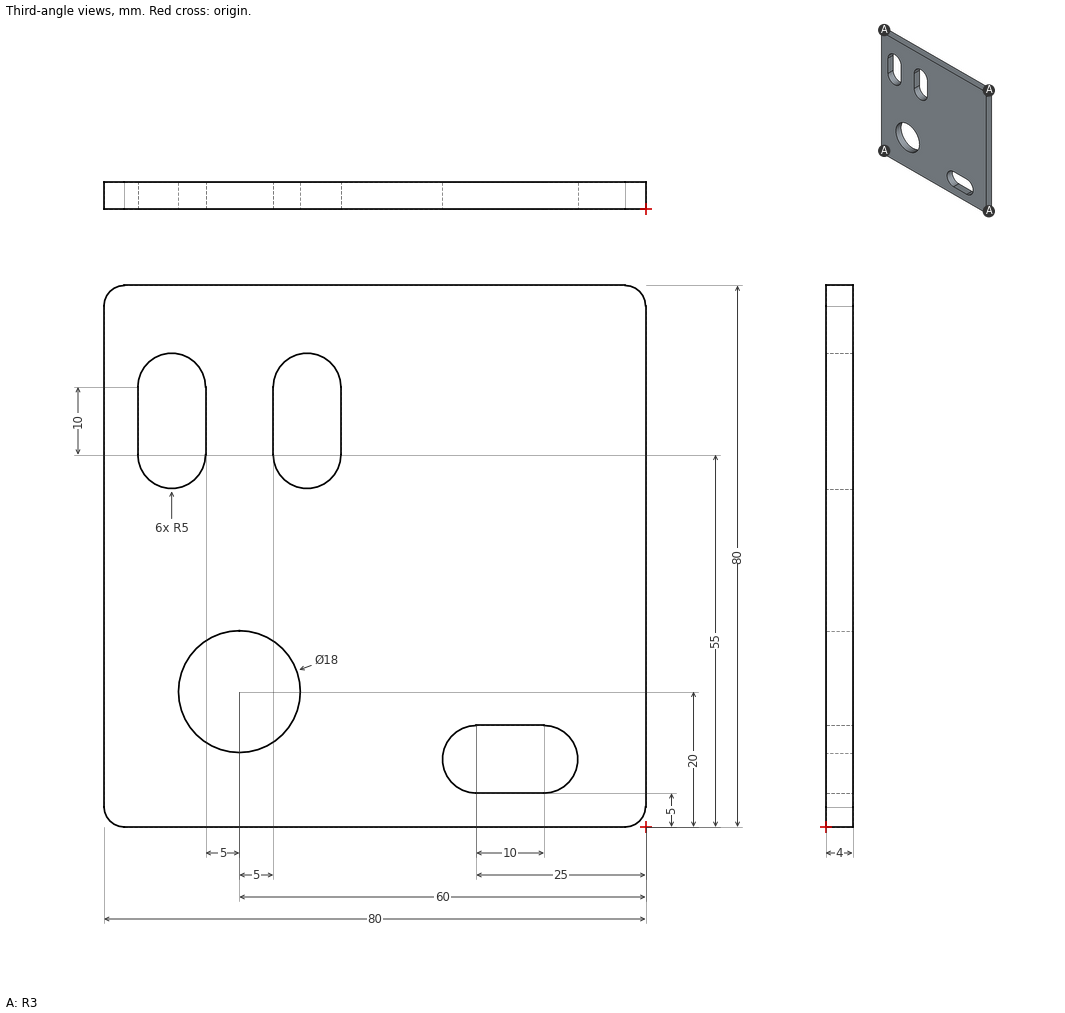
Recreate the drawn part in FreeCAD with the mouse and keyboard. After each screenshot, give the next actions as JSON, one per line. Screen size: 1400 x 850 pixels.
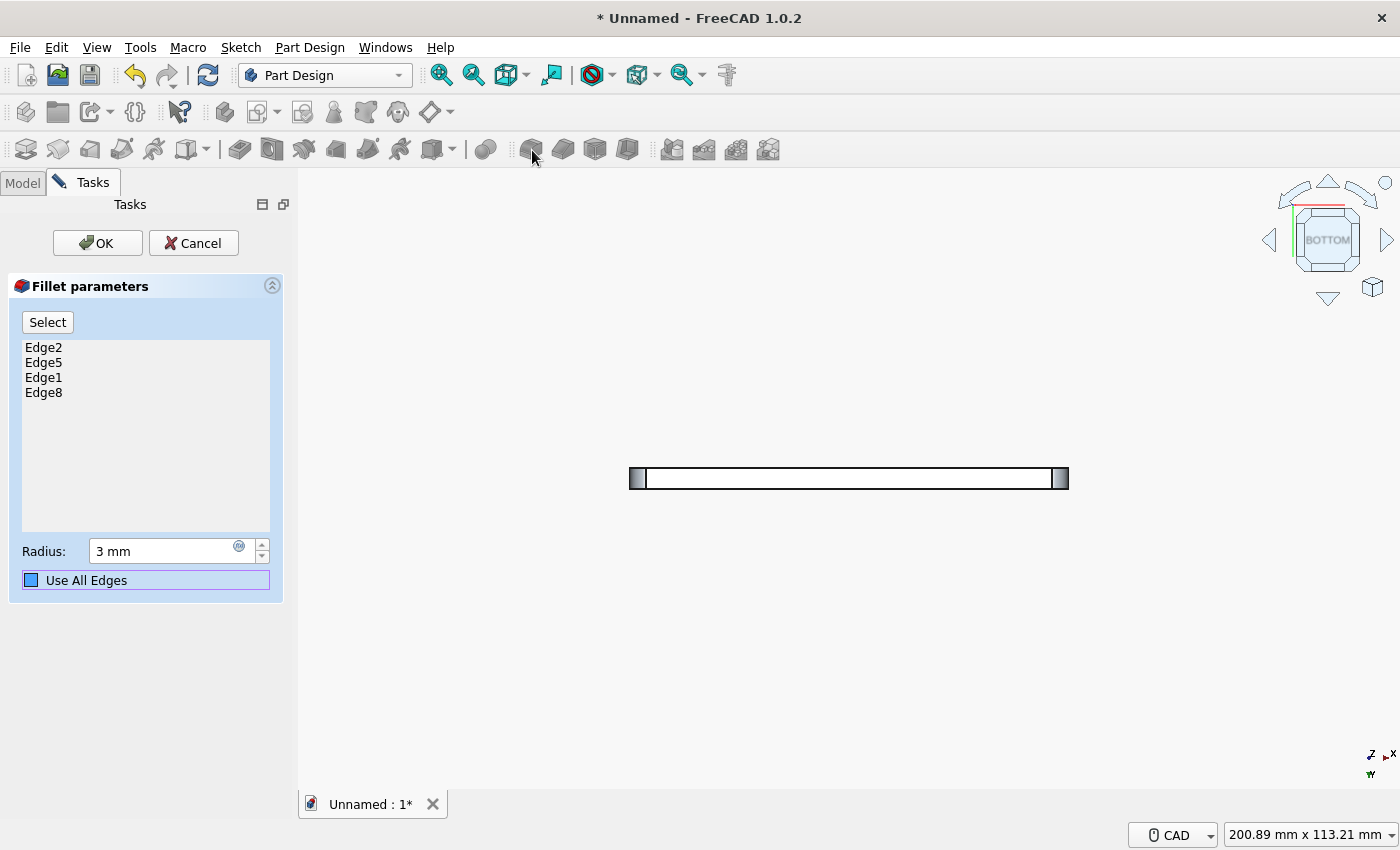
{"action": "left_click", "coordinate": [98, 243]}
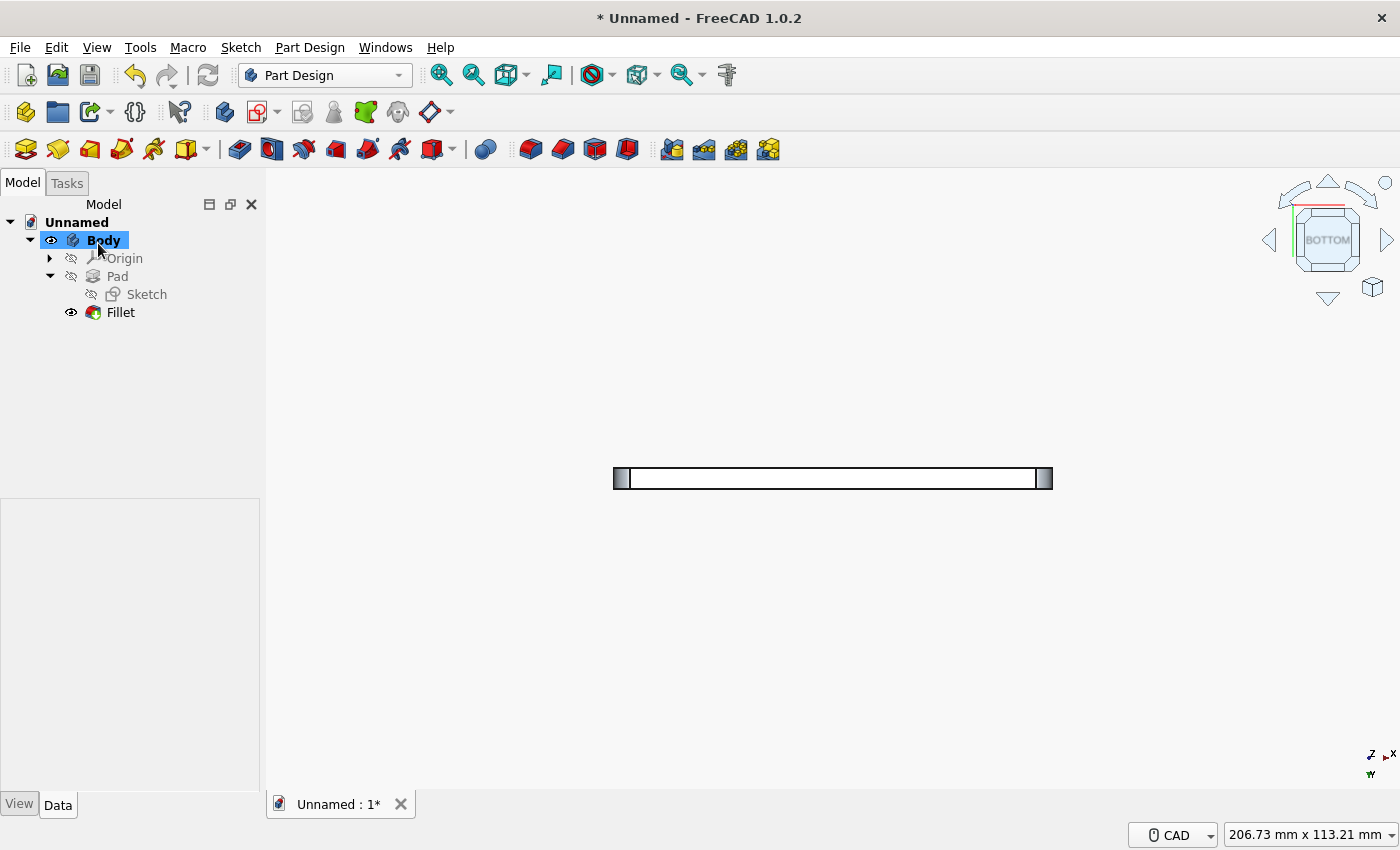
{"action": "key", "text": "0"}